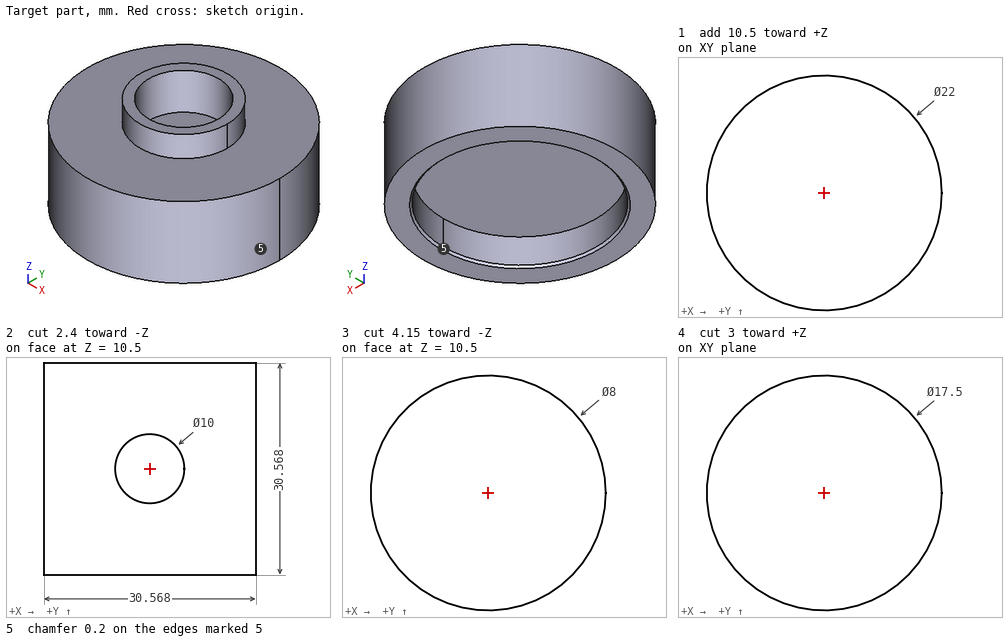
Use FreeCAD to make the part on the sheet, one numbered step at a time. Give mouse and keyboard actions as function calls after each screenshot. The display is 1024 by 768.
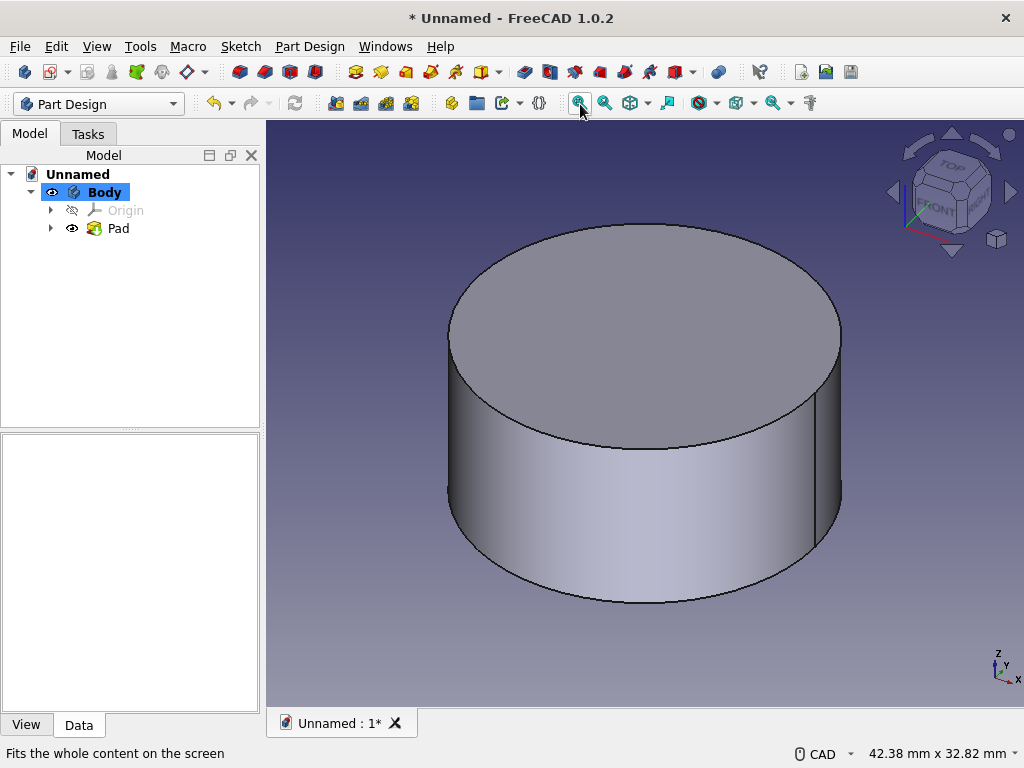
click(645, 336)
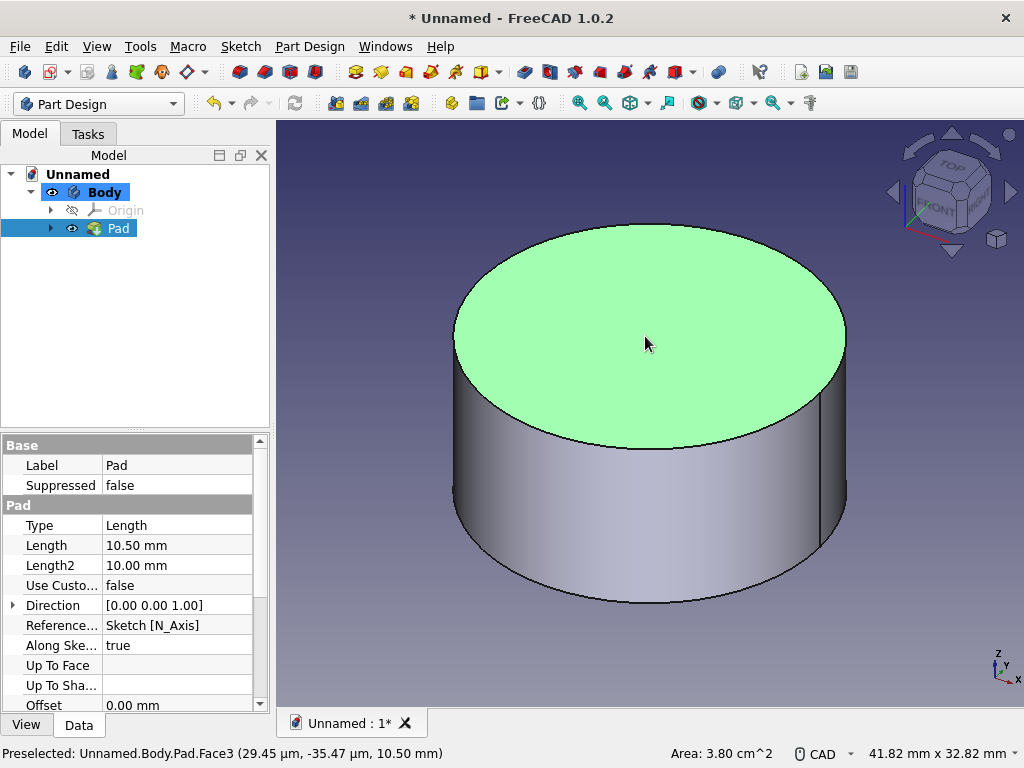
click(50, 72)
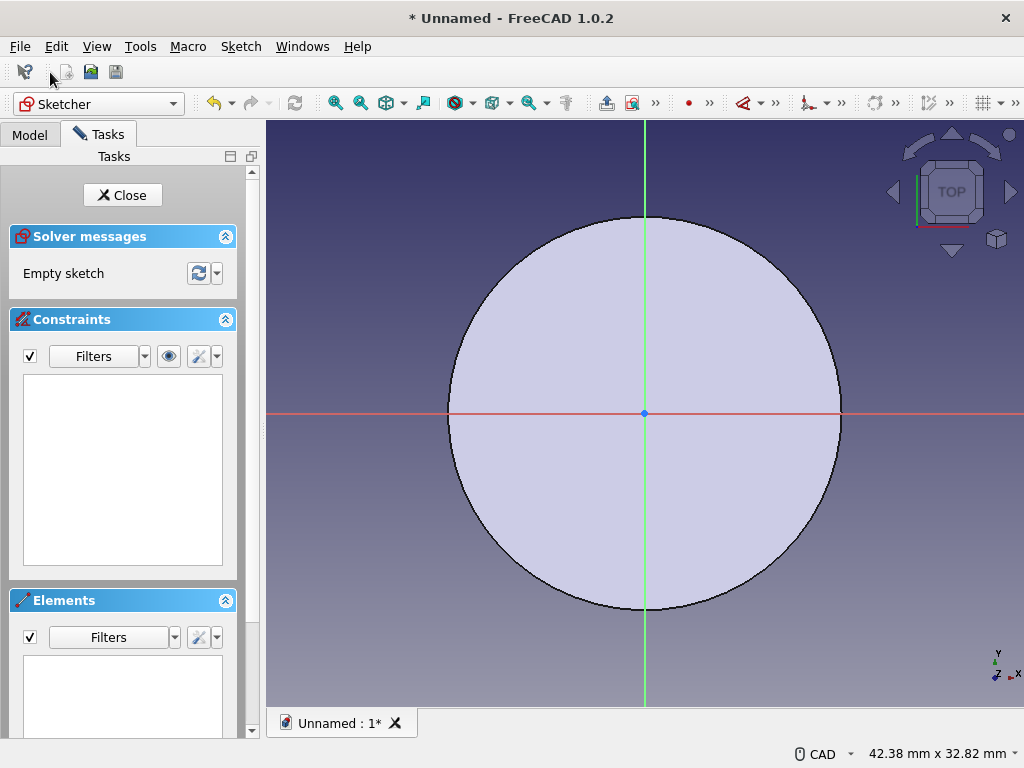
scroll(438, 414, down, 2)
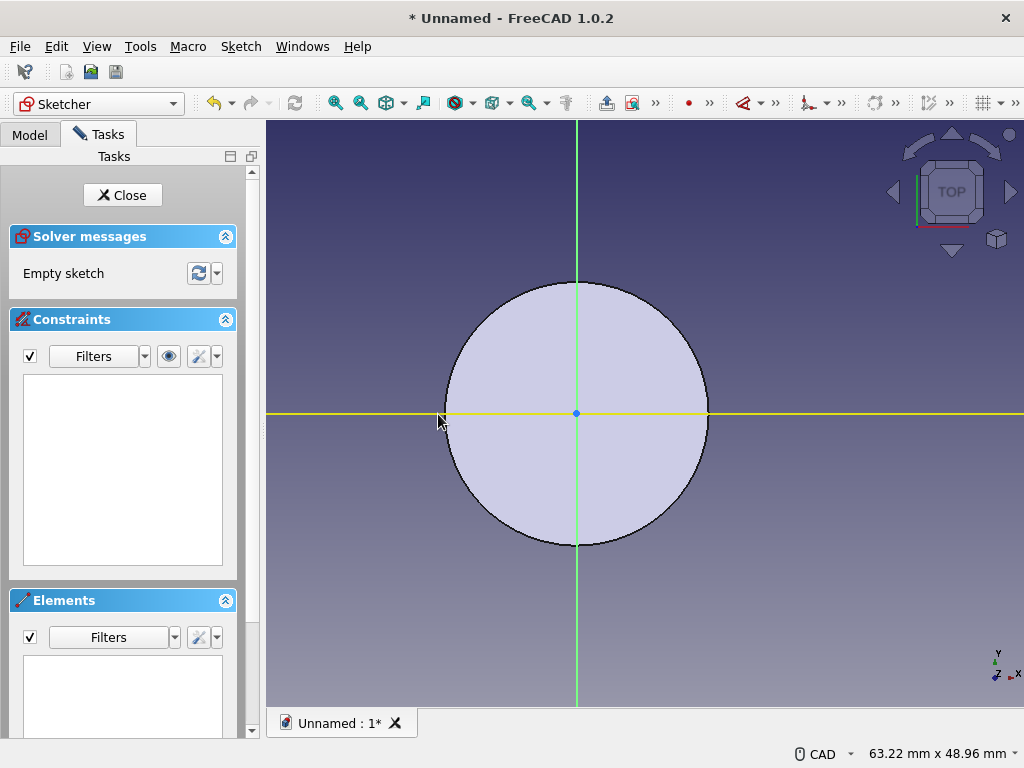
key(g)
key(v)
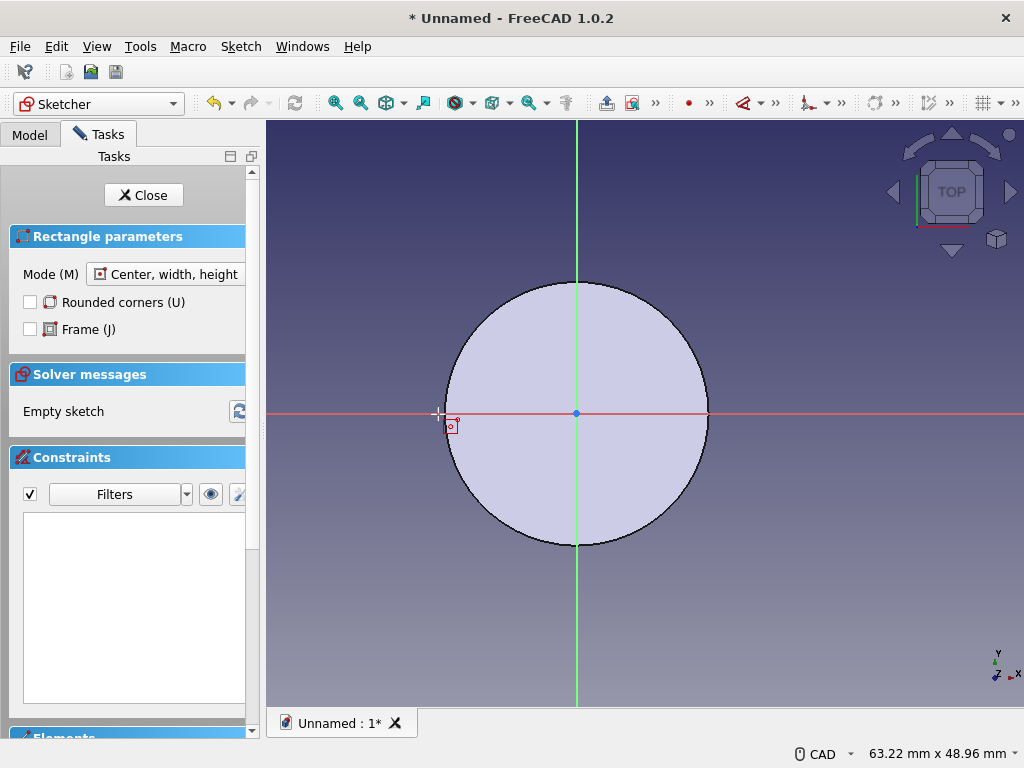
click(577, 414)
move(760, 231)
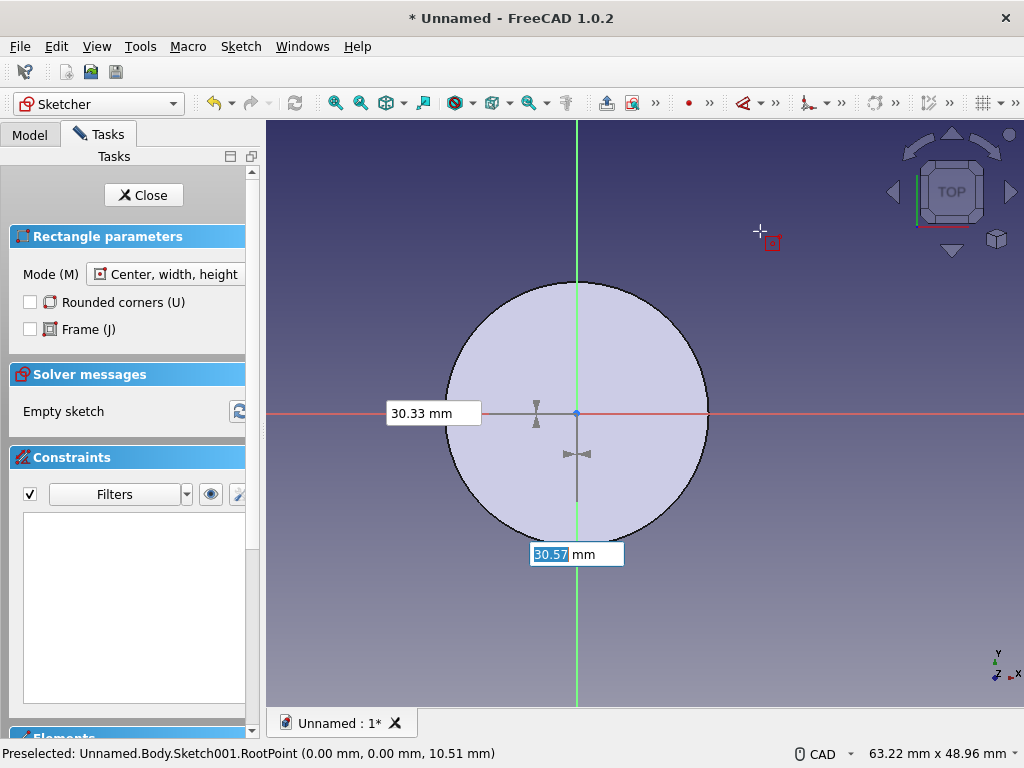
text(30.568)
key(Tab)
text(30.568)
key(Return)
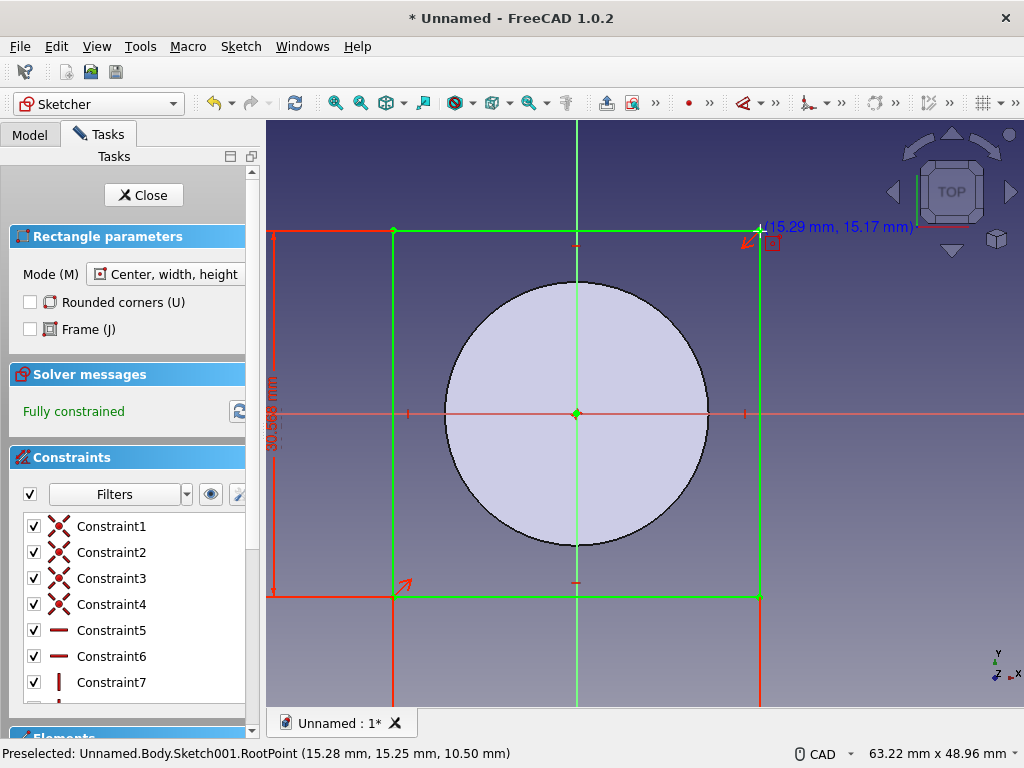
key(g)
key(c)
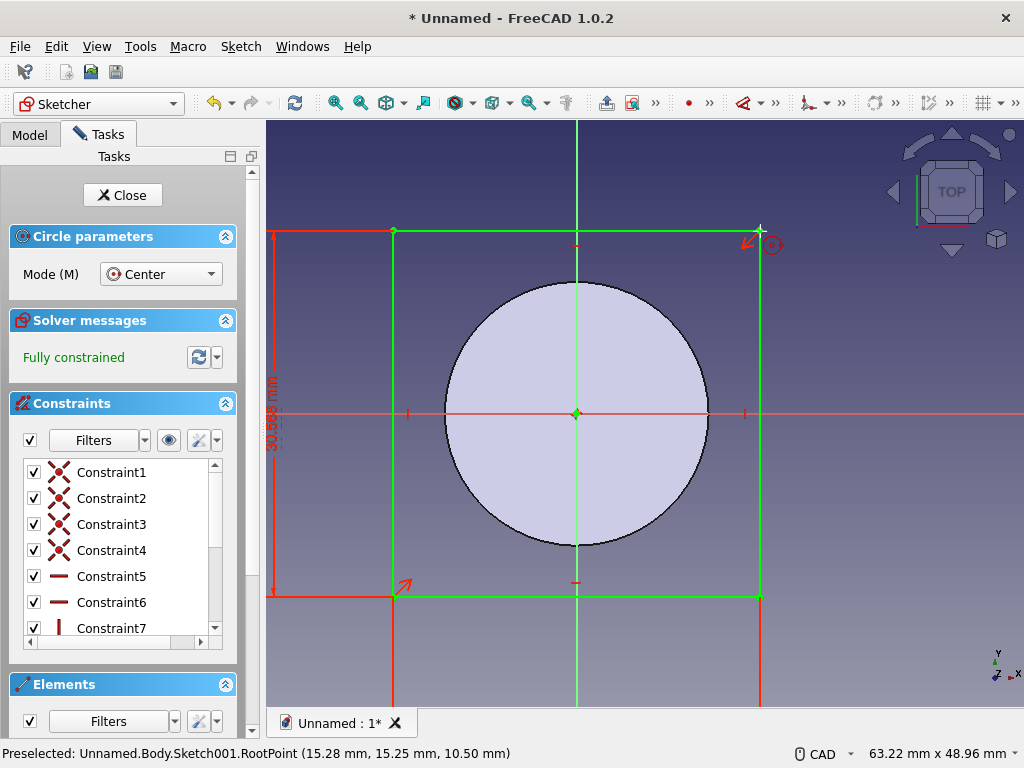
click(577, 414)
move(619, 371)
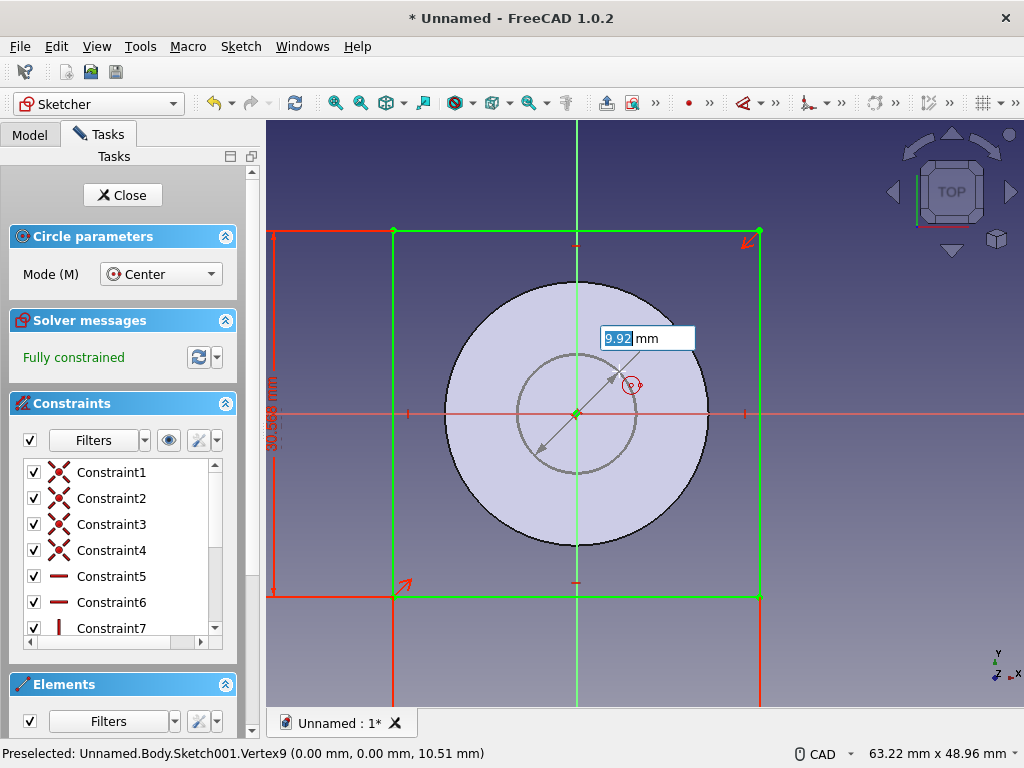
text(10)
key(Return)
key(Escape)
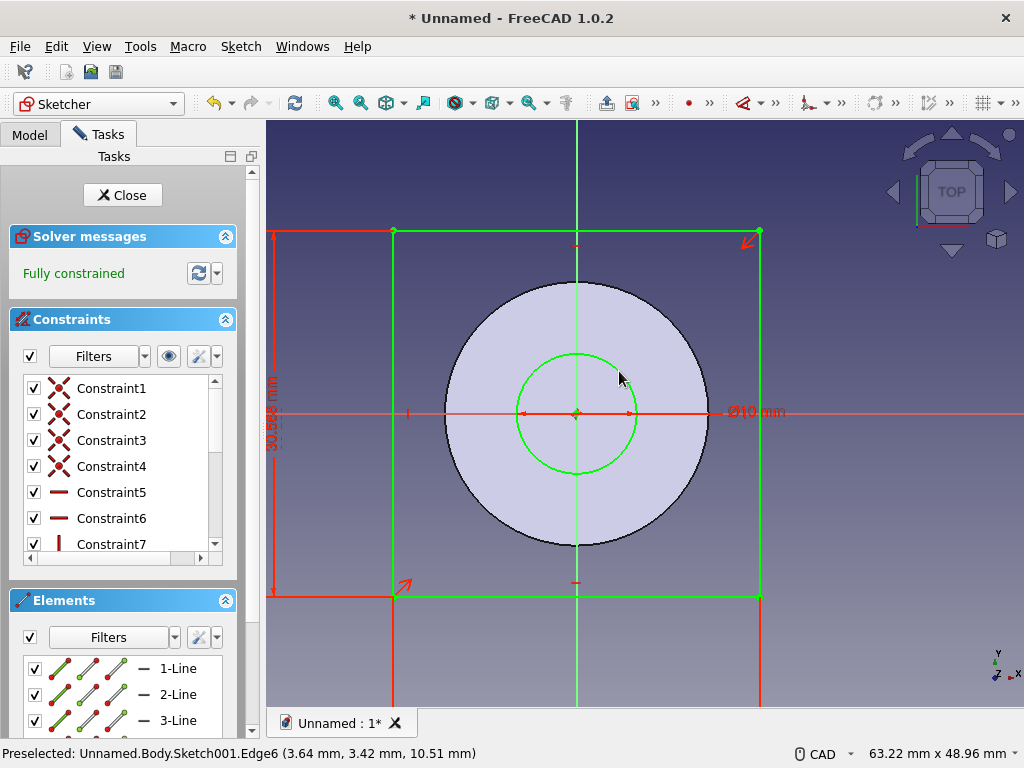
click(123, 195)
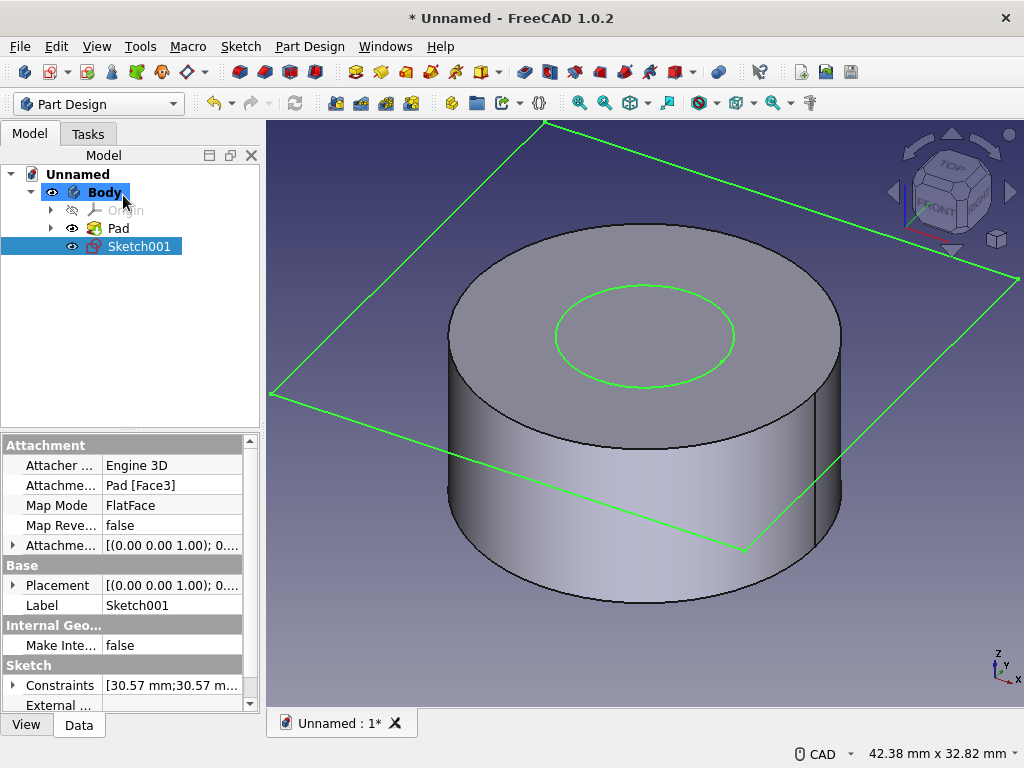
click(525, 72)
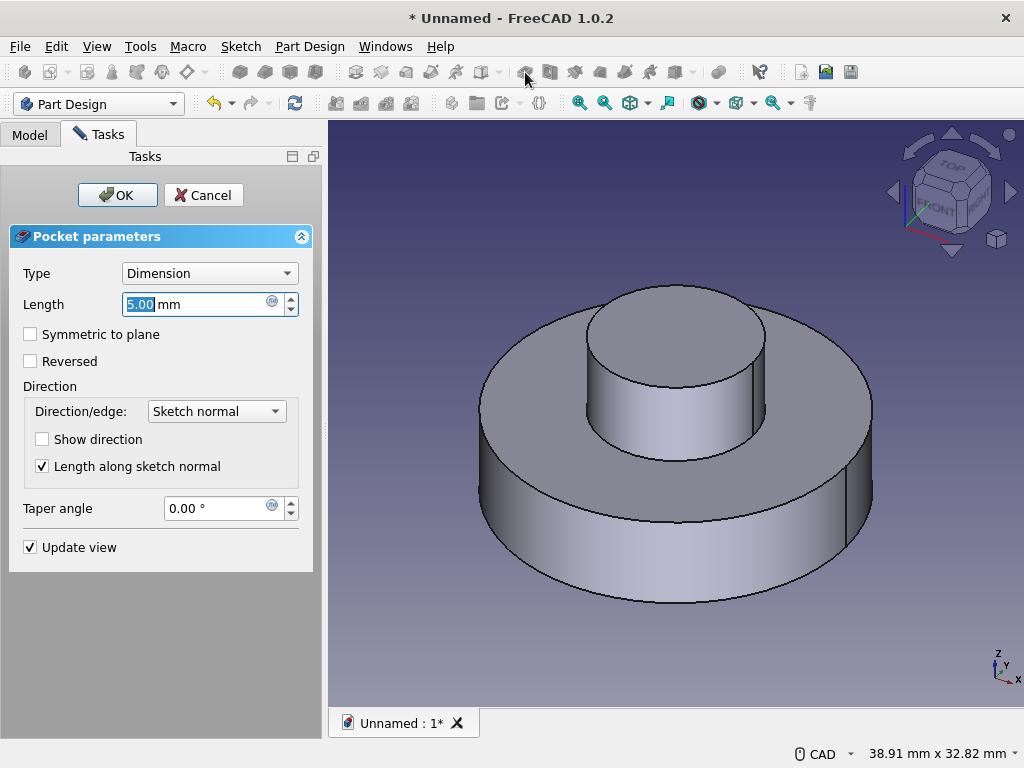
text(2.4)
key(Tab)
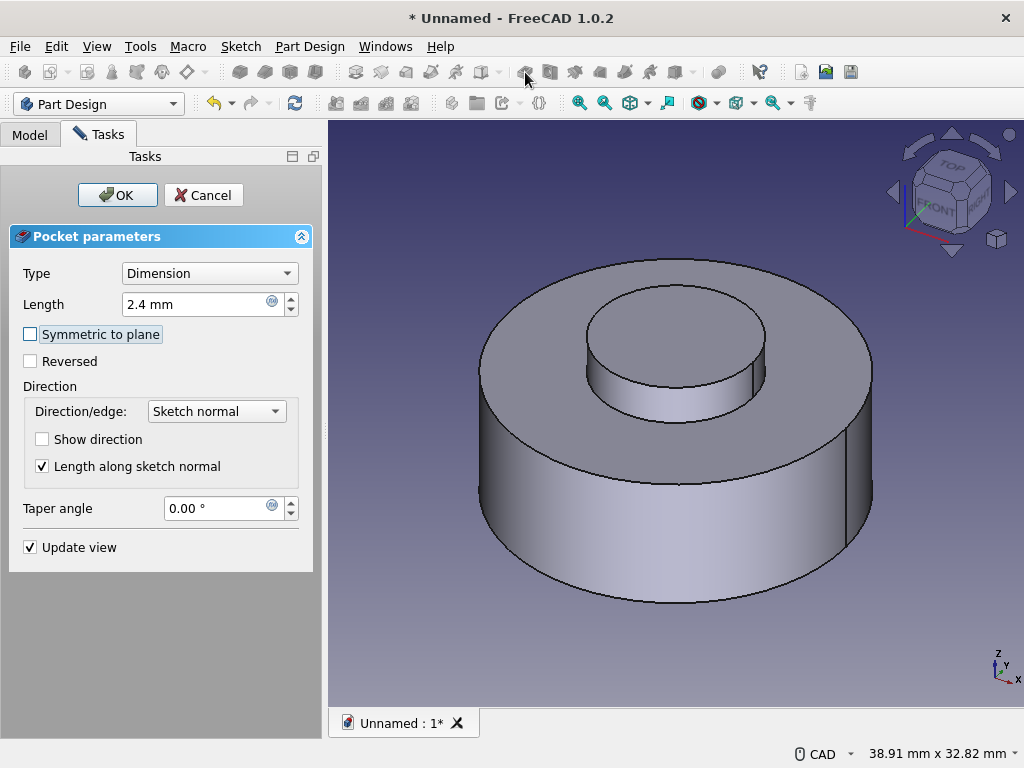
click(118, 195)